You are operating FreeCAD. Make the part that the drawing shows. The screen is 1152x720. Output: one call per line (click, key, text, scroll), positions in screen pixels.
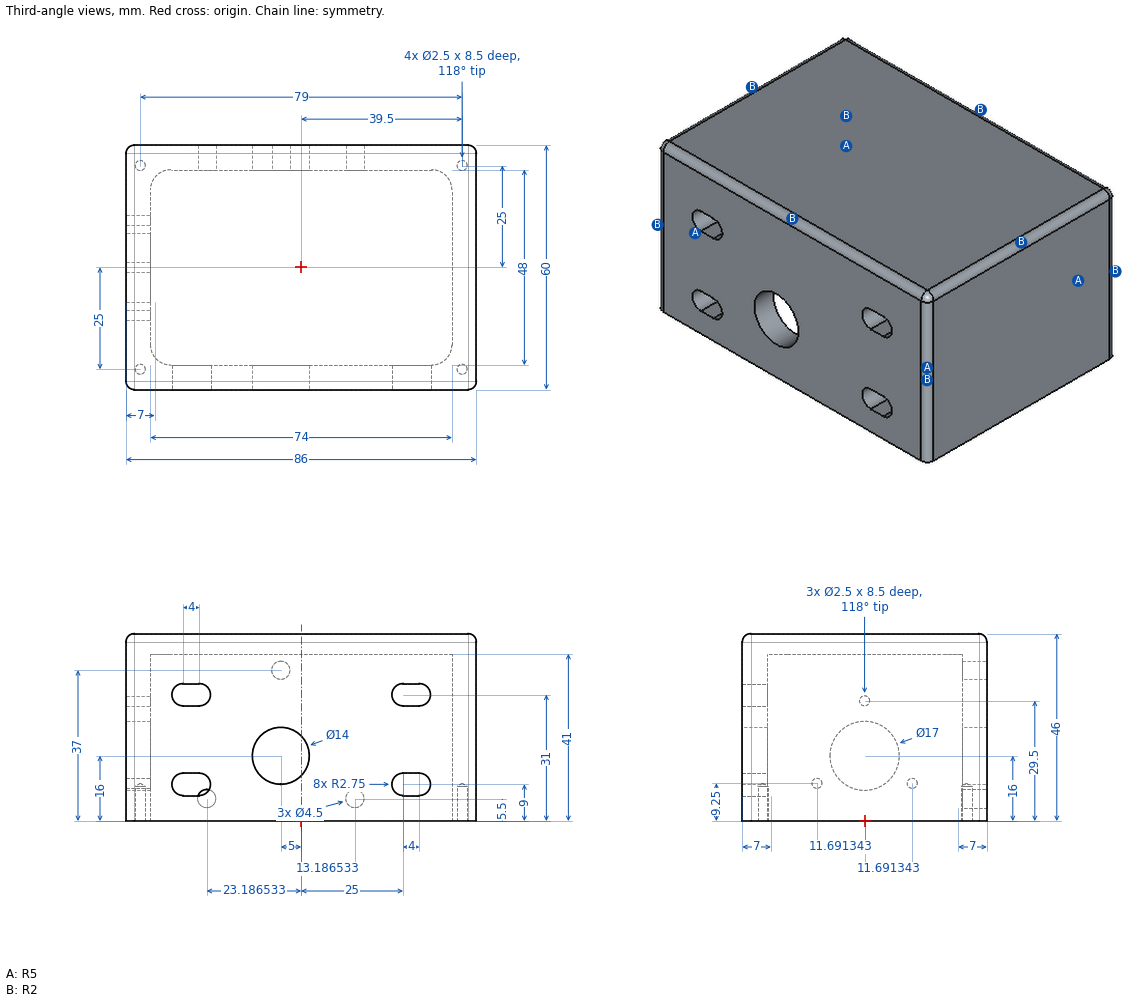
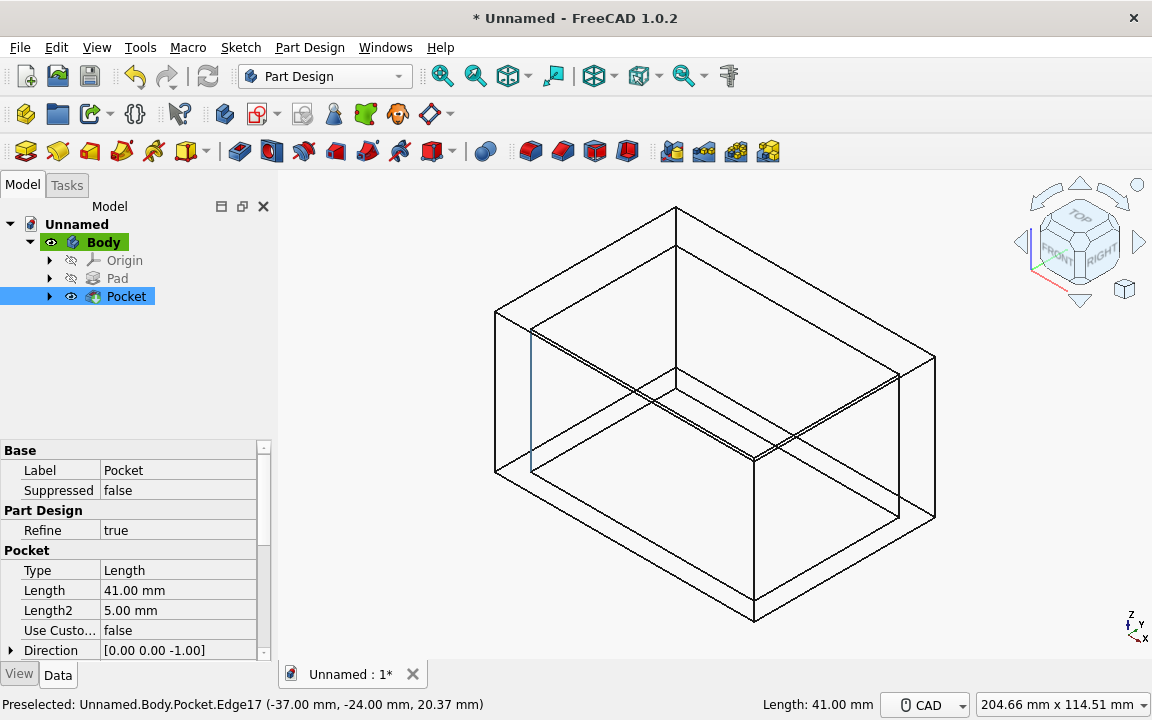
click(899, 445, ctrl)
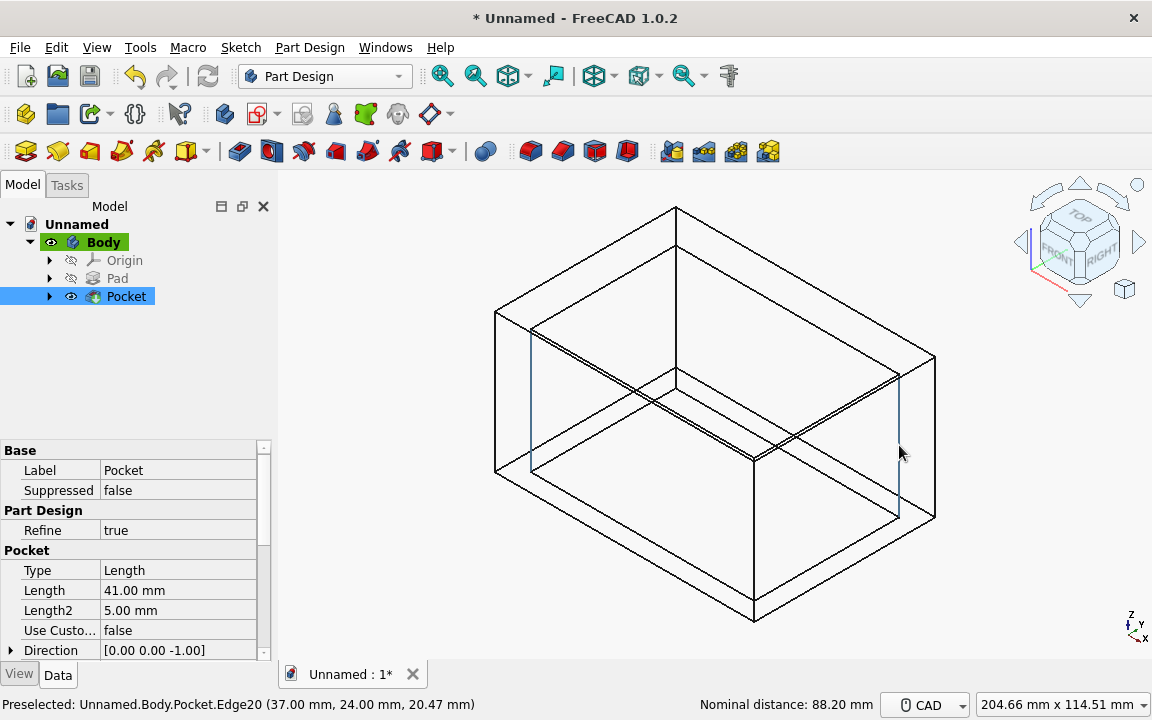
click(676, 316, ctrl)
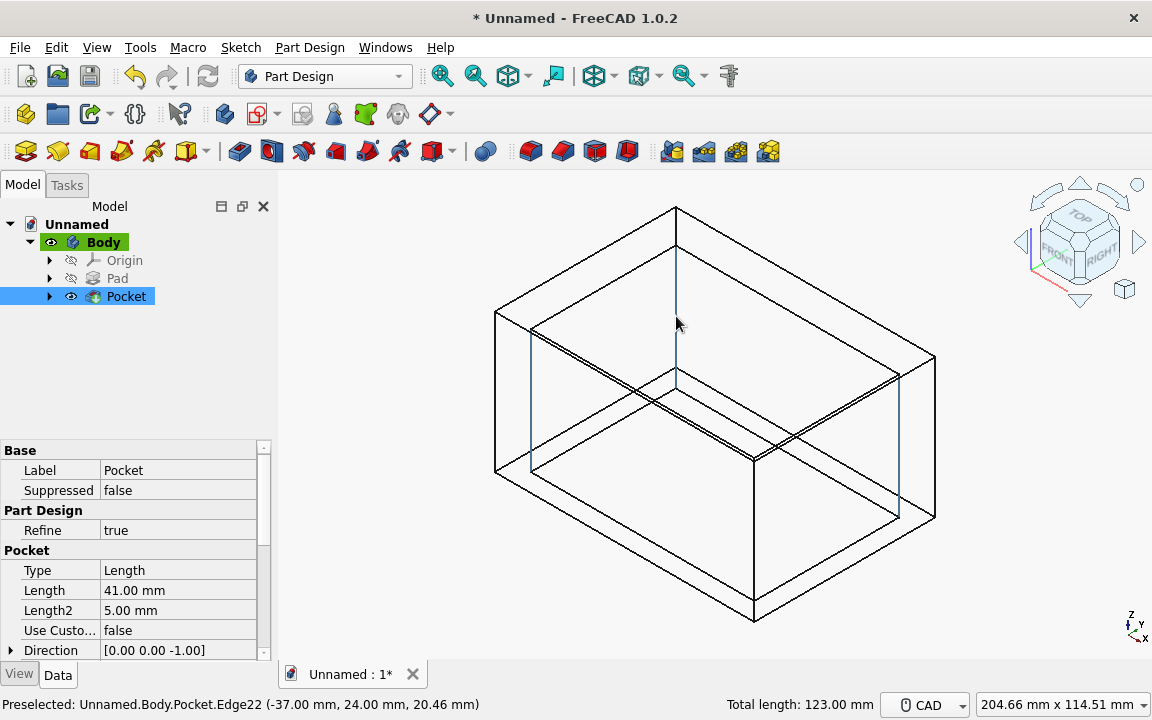
key(2)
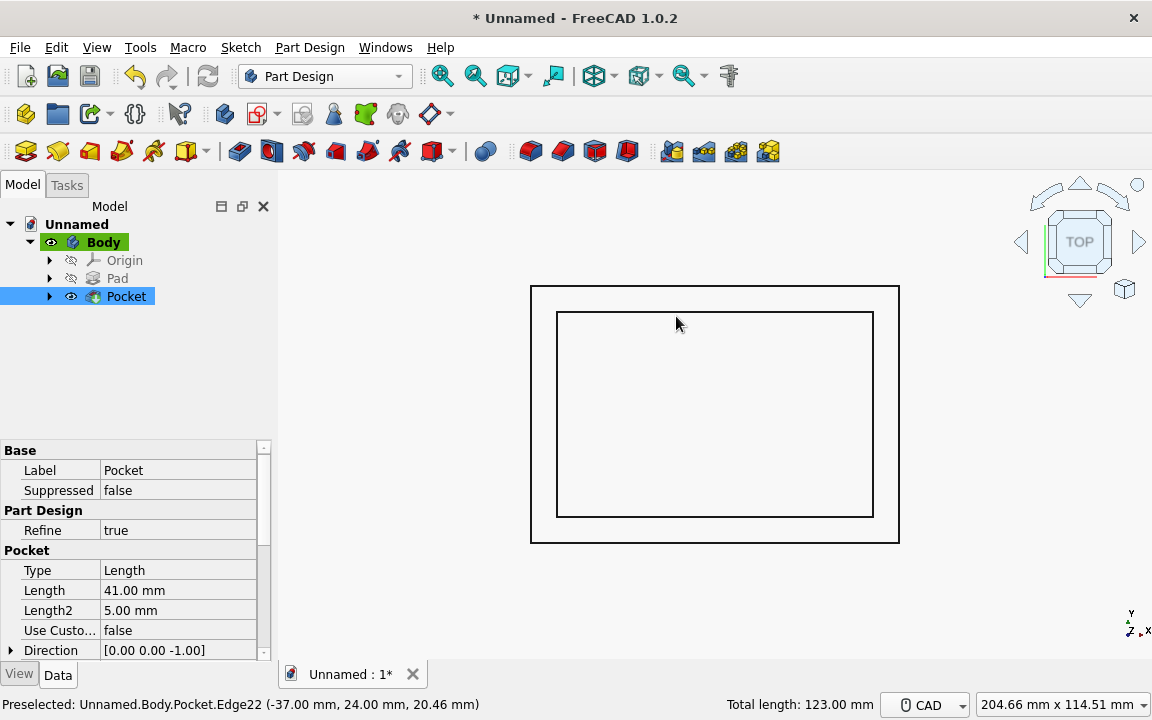
key(1)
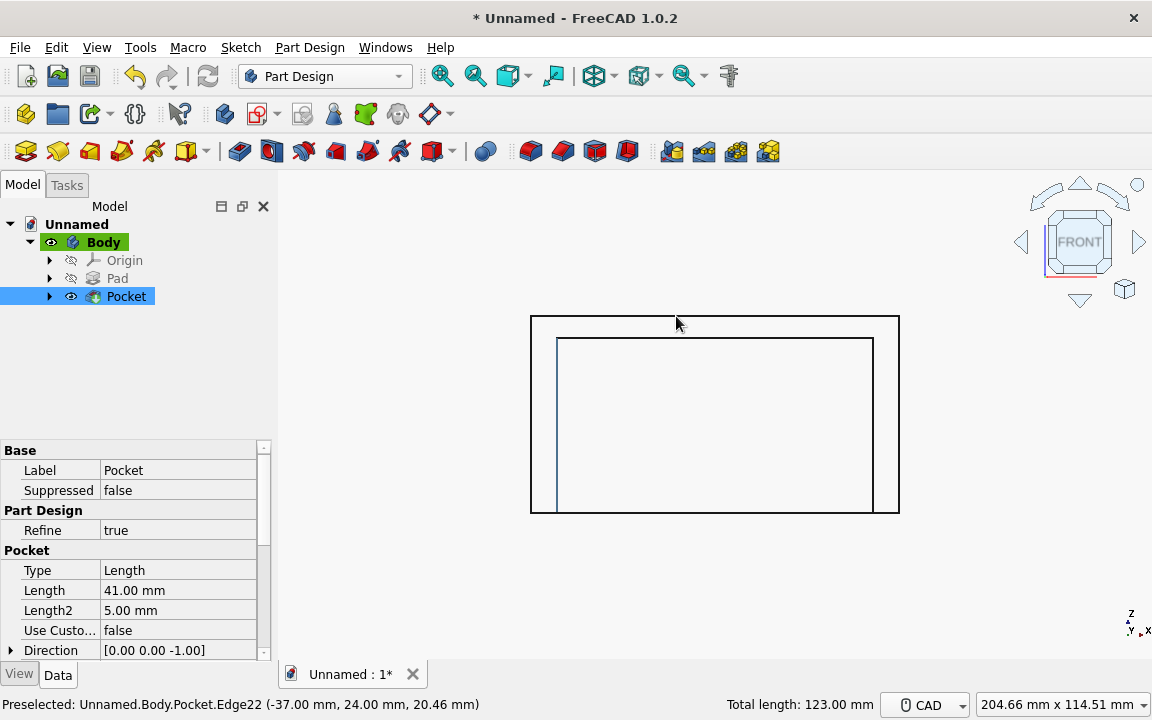
key(v)
key(f)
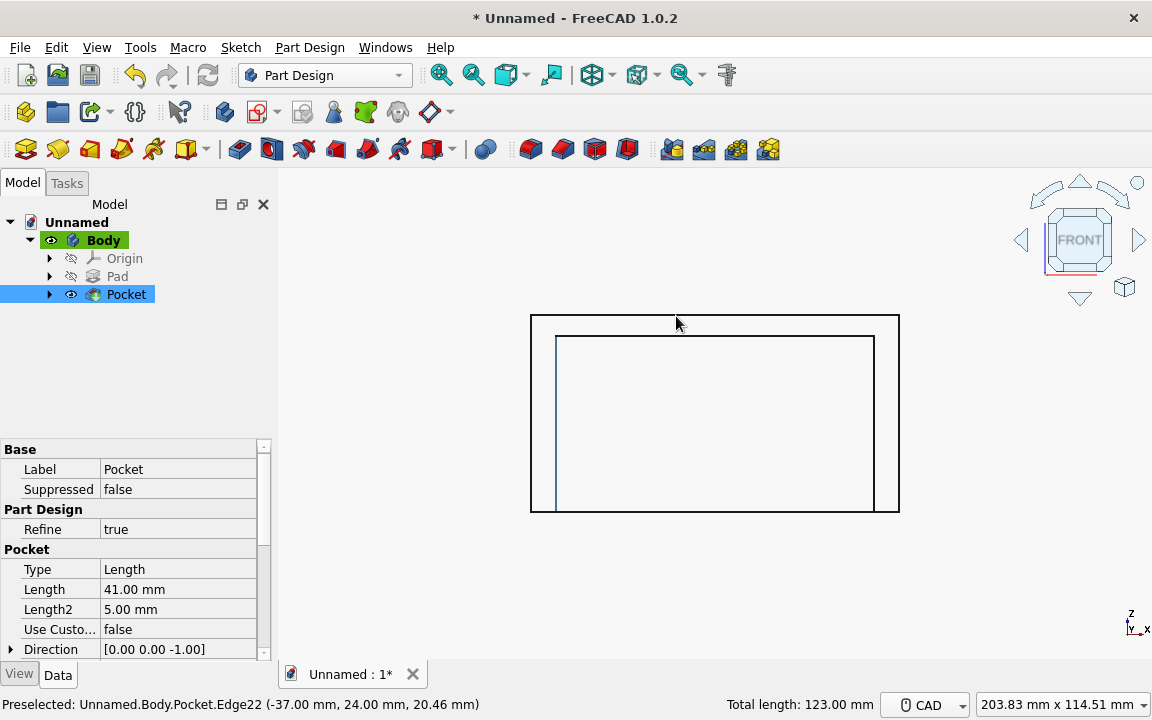
click(874, 423, ctrl)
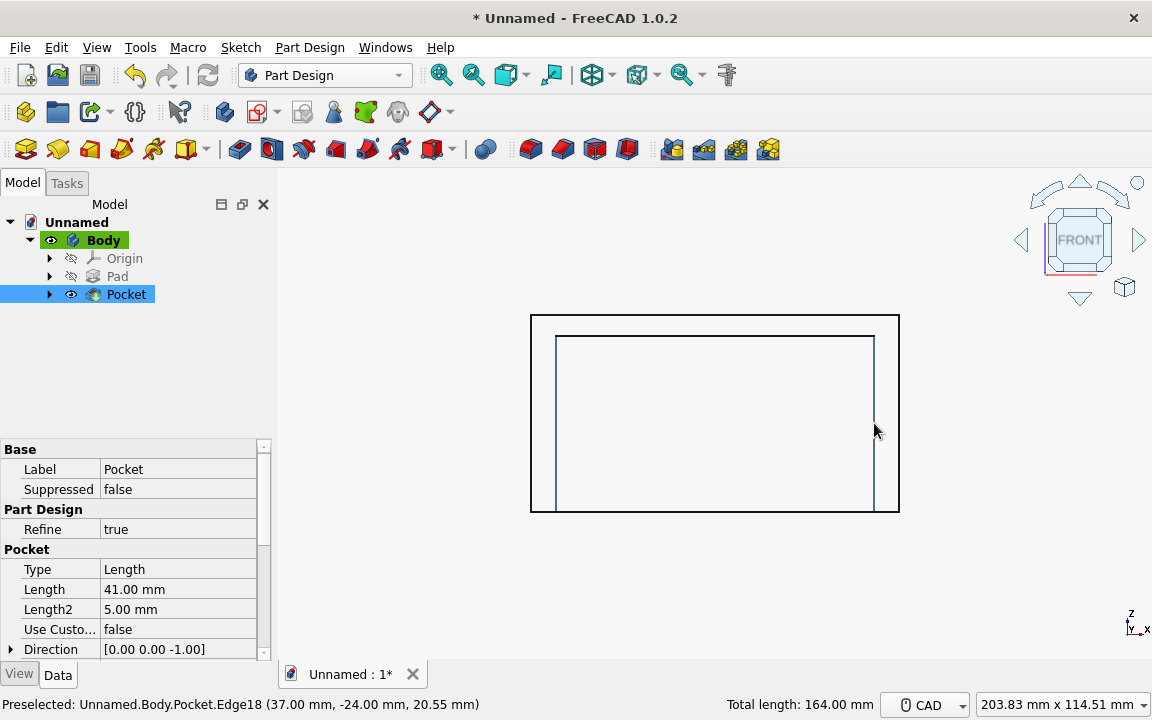
key(v)
key(1)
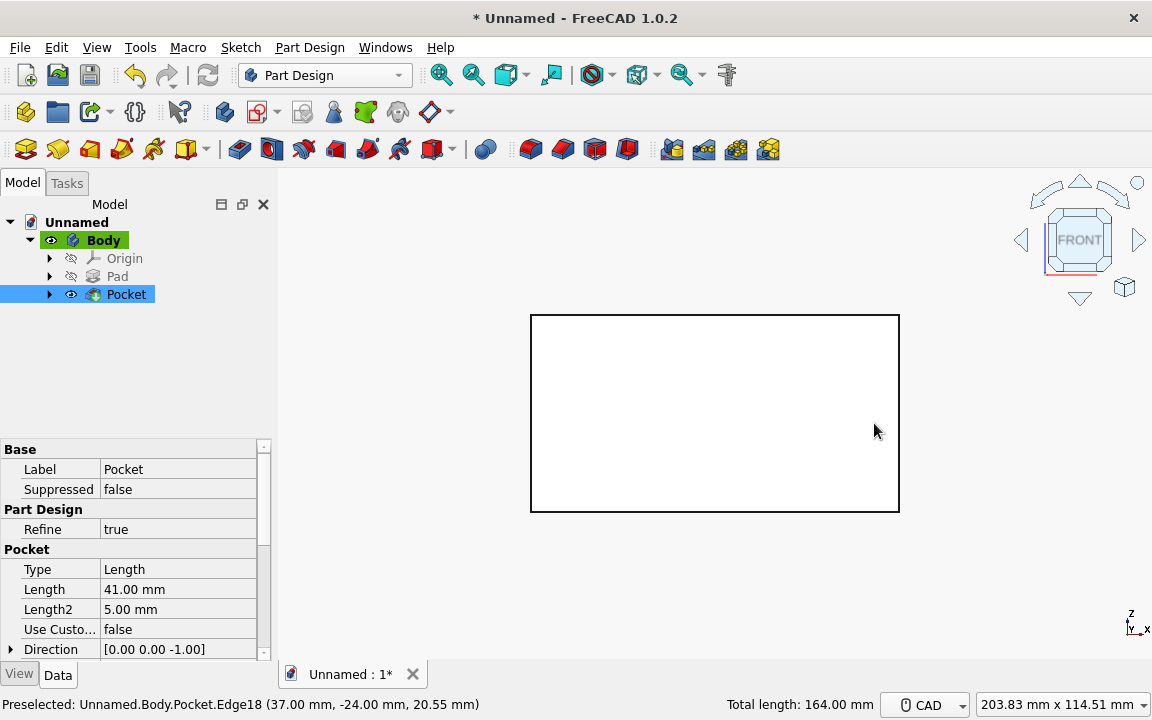
click(532, 150)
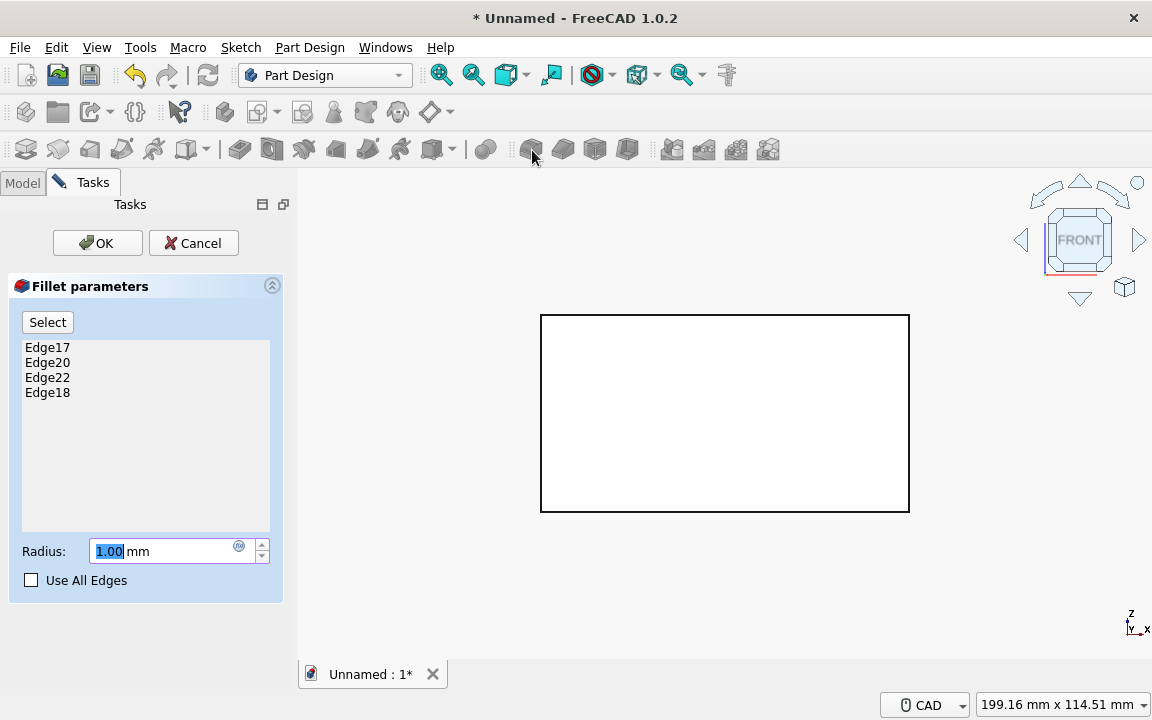
text(5)
key(Tab)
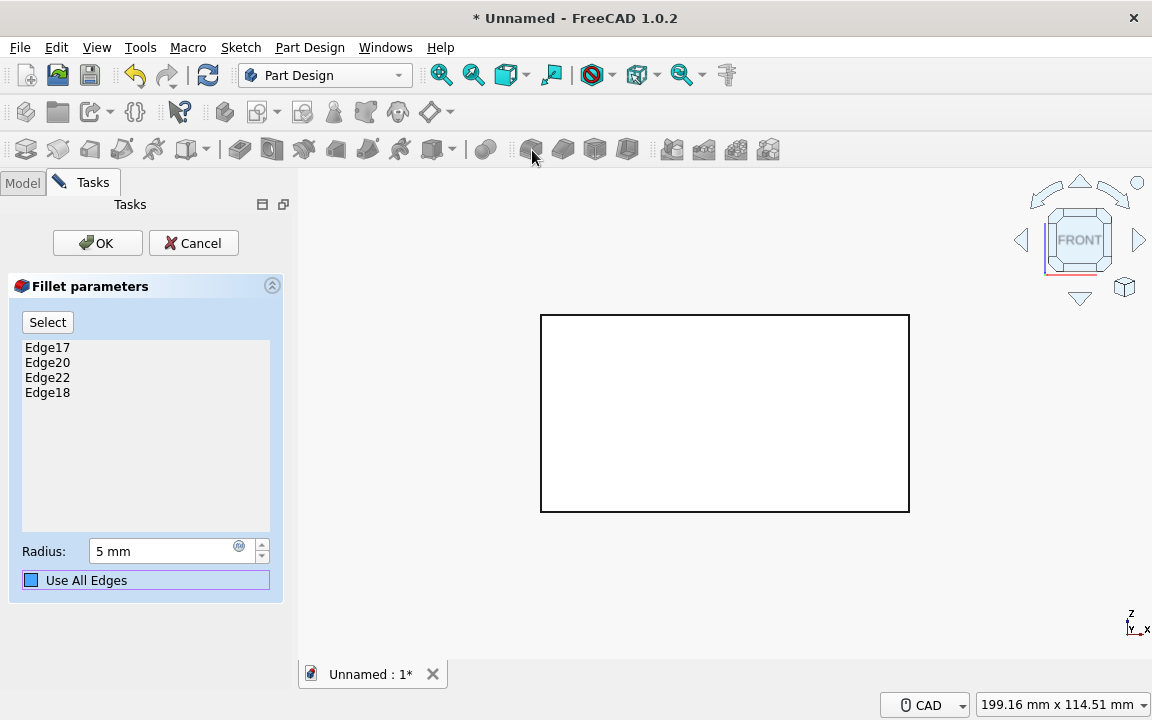
click(98, 243)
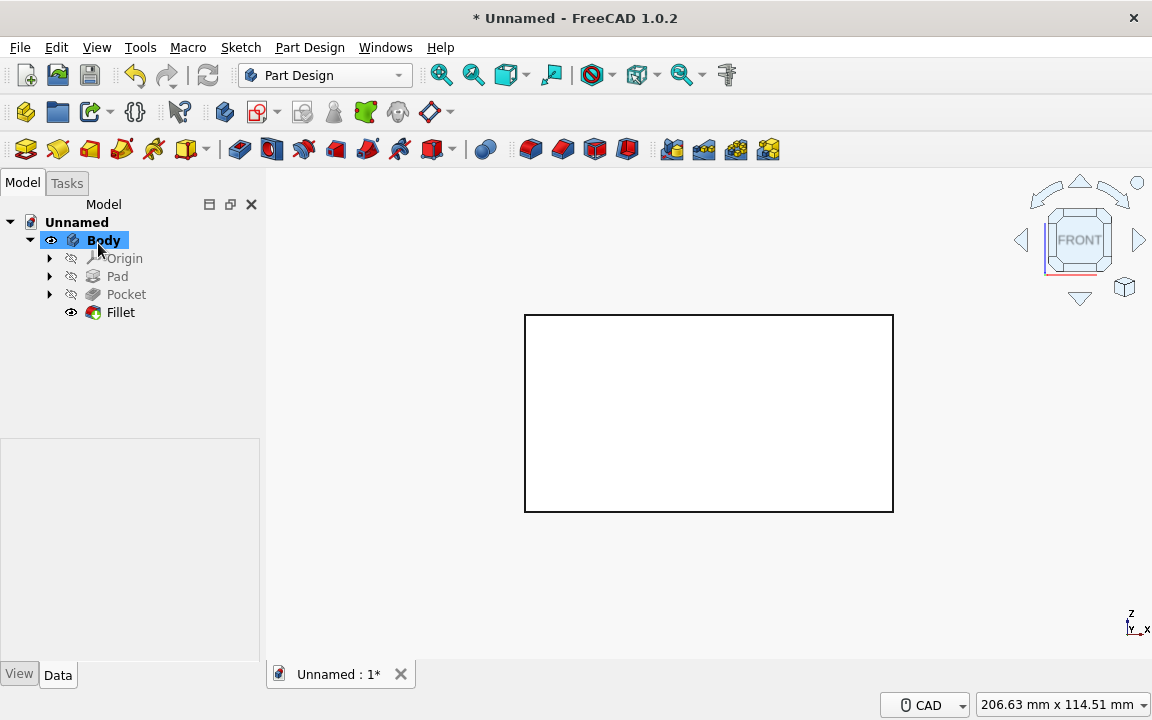
key(v)
key(f)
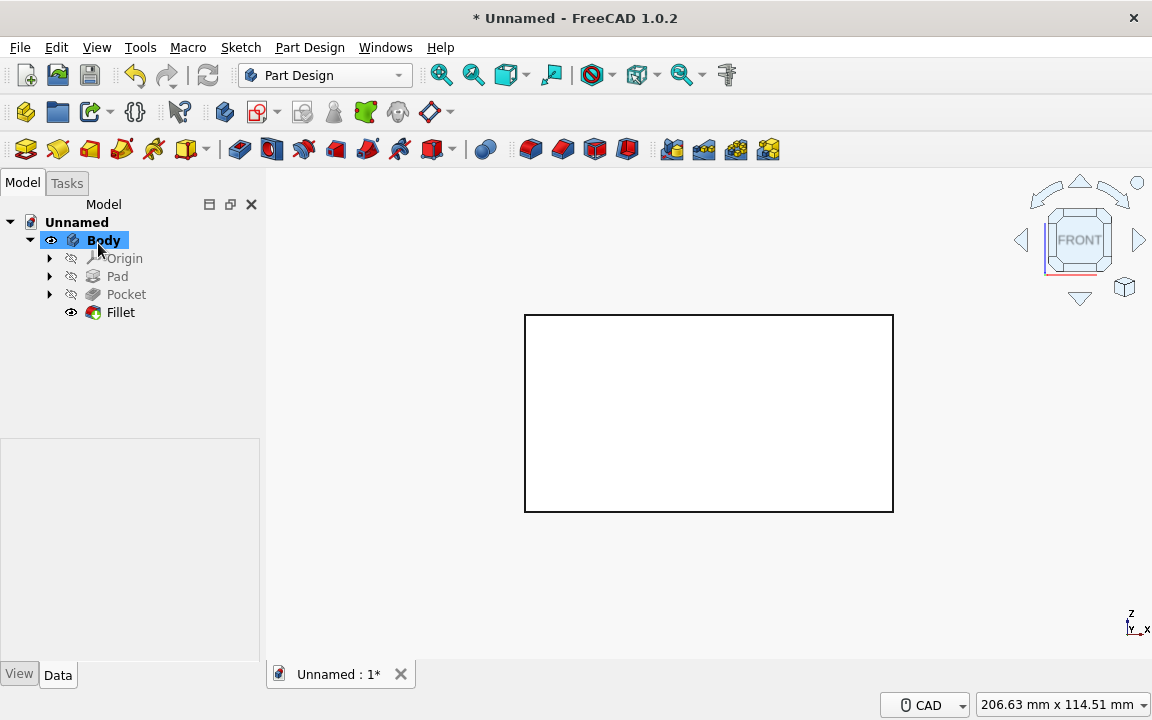
click(762, 413)